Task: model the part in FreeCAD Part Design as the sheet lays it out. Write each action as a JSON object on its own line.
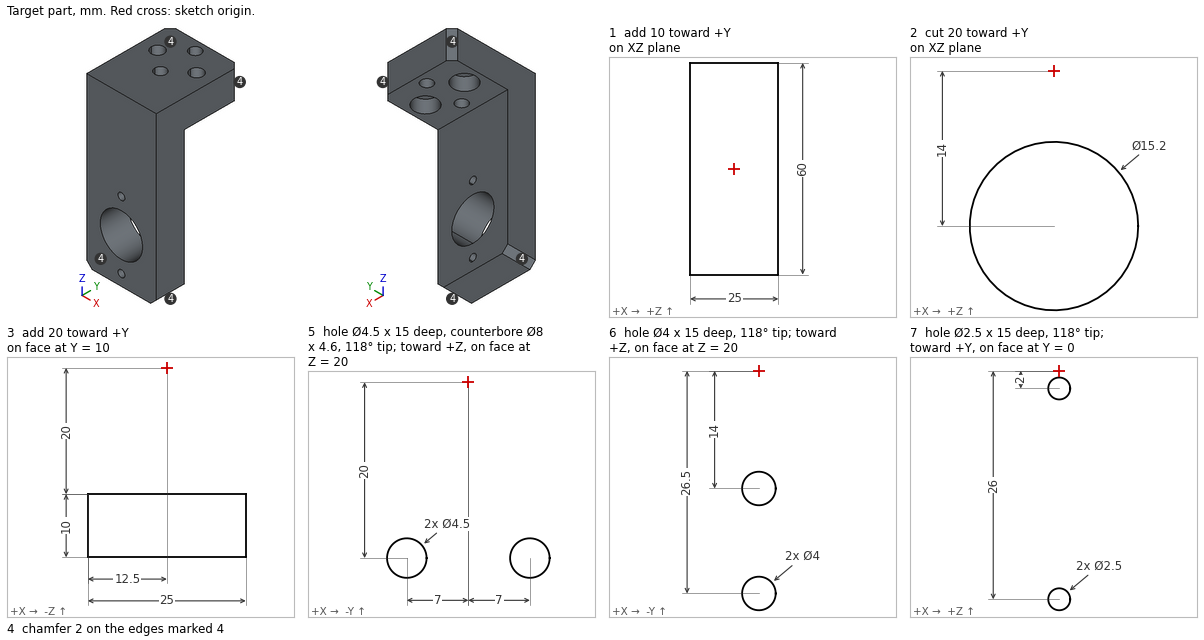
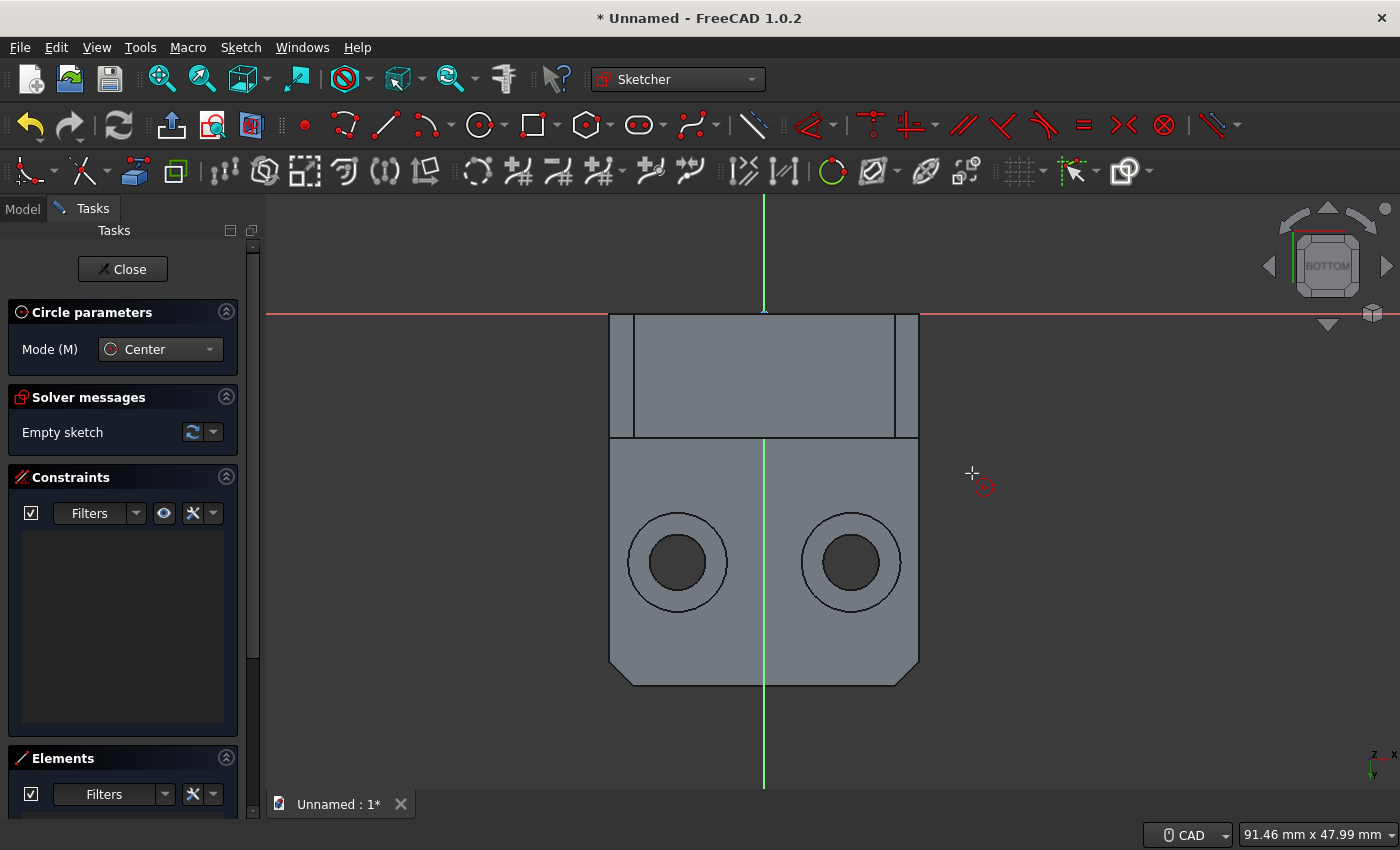
{"action": "left_click", "coordinate": [764, 643]}
{"action": "left_click", "coordinate": [782, 625]}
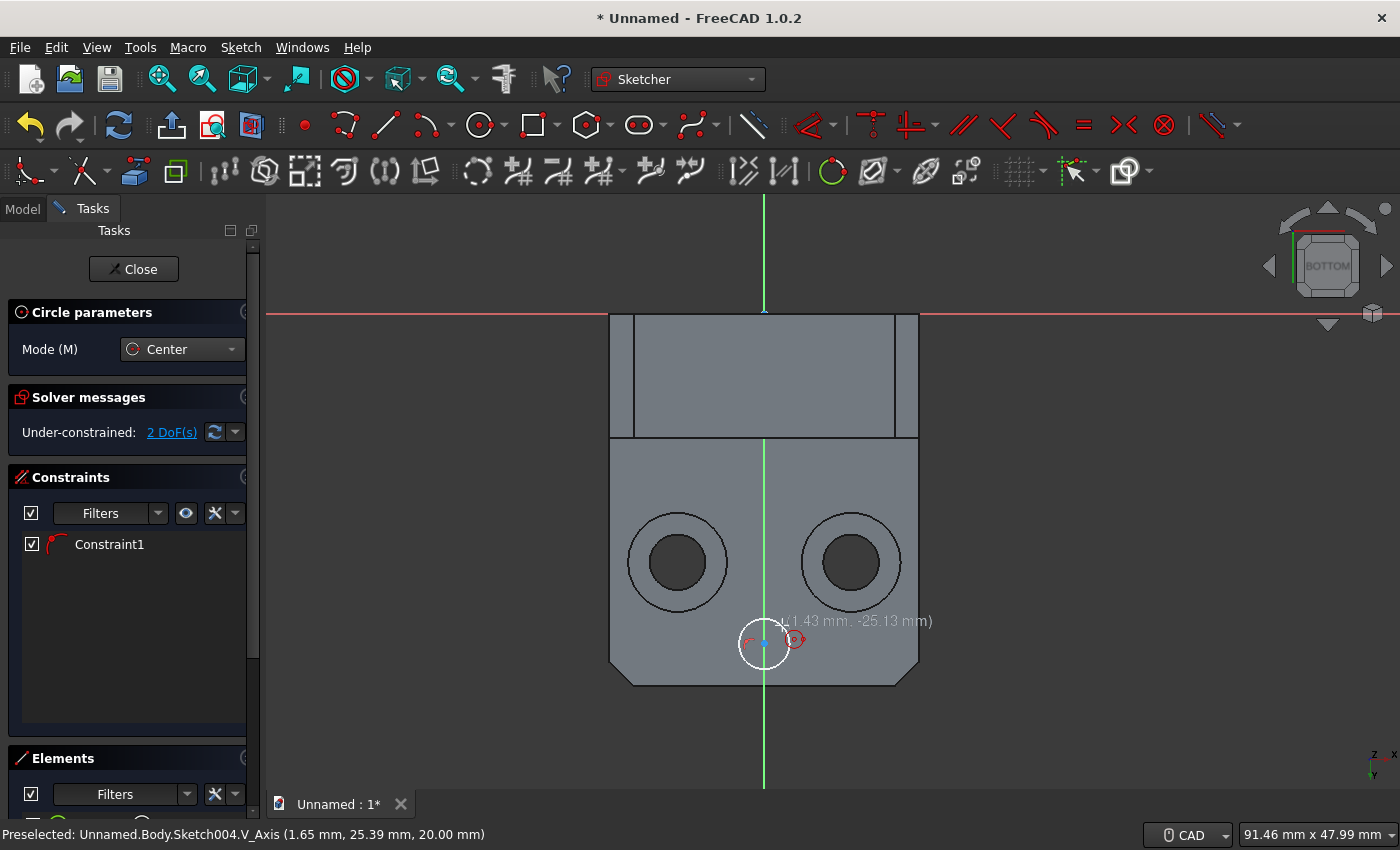
{"action": "left_click", "coordinate": [764, 488]}
{"action": "left_click", "coordinate": [782, 470]}
{"action": "key", "text": "Escape"}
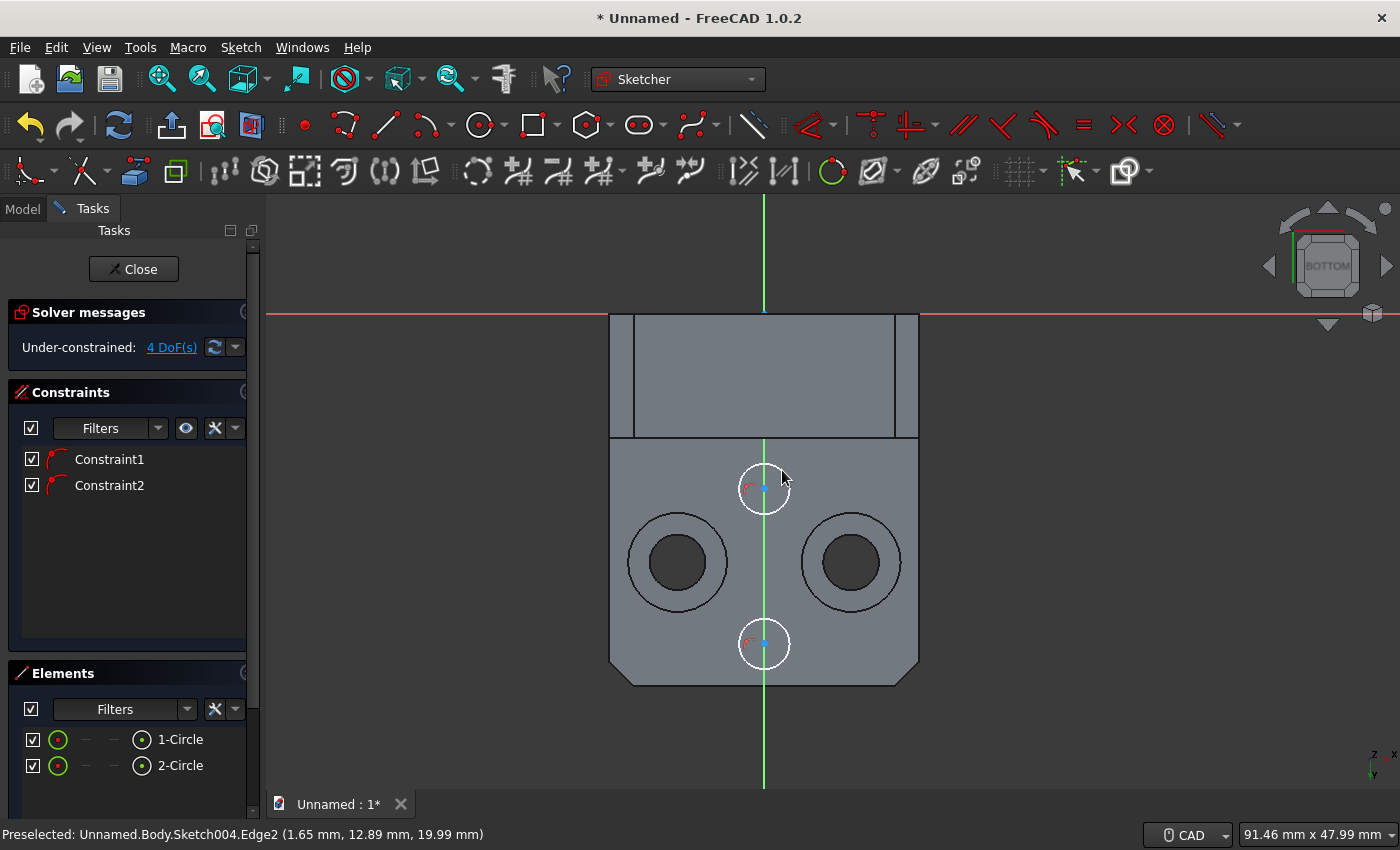
{"action": "left_click", "coordinate": [782, 626]}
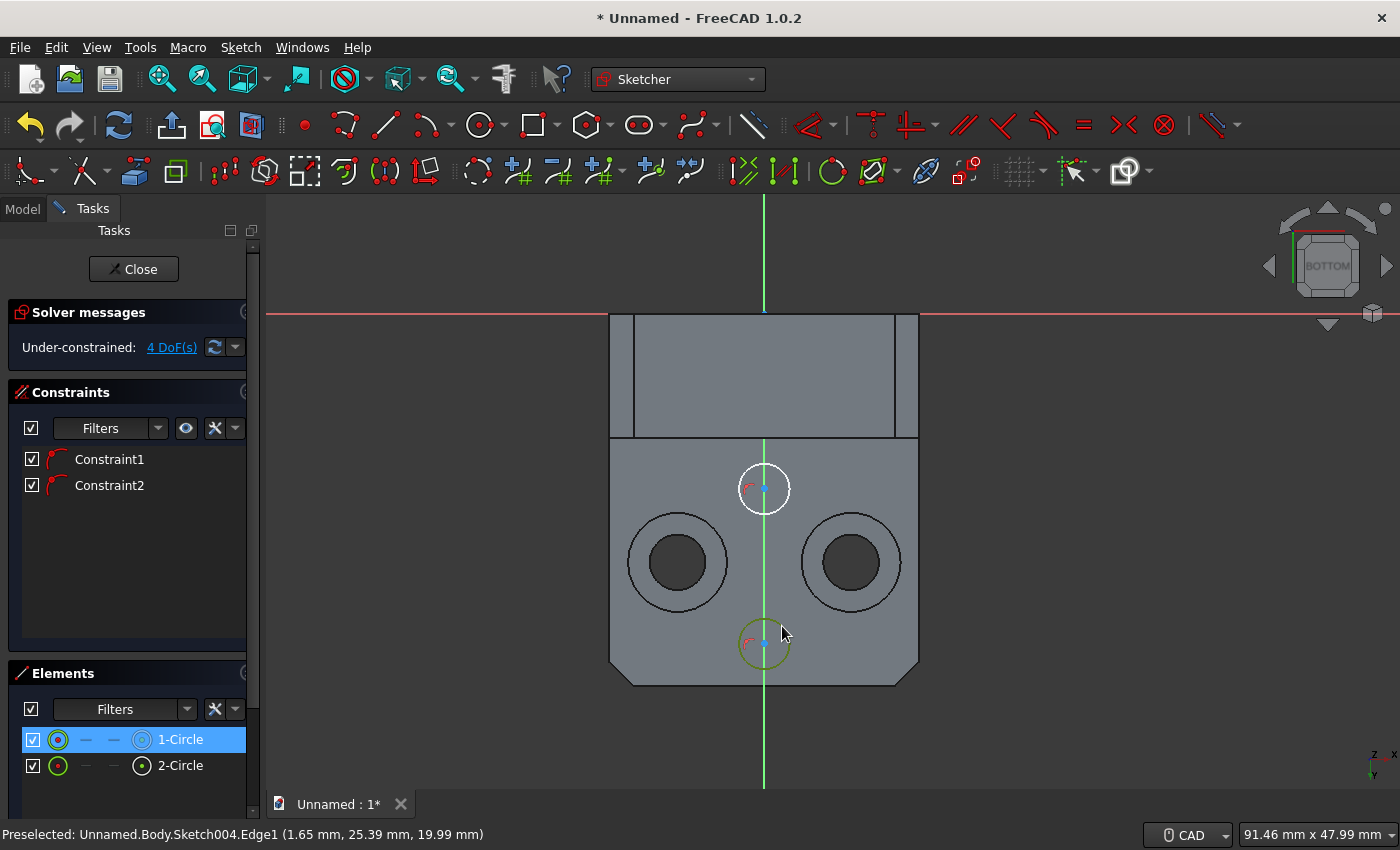
{"action": "left_click", "coordinate": [782, 471]}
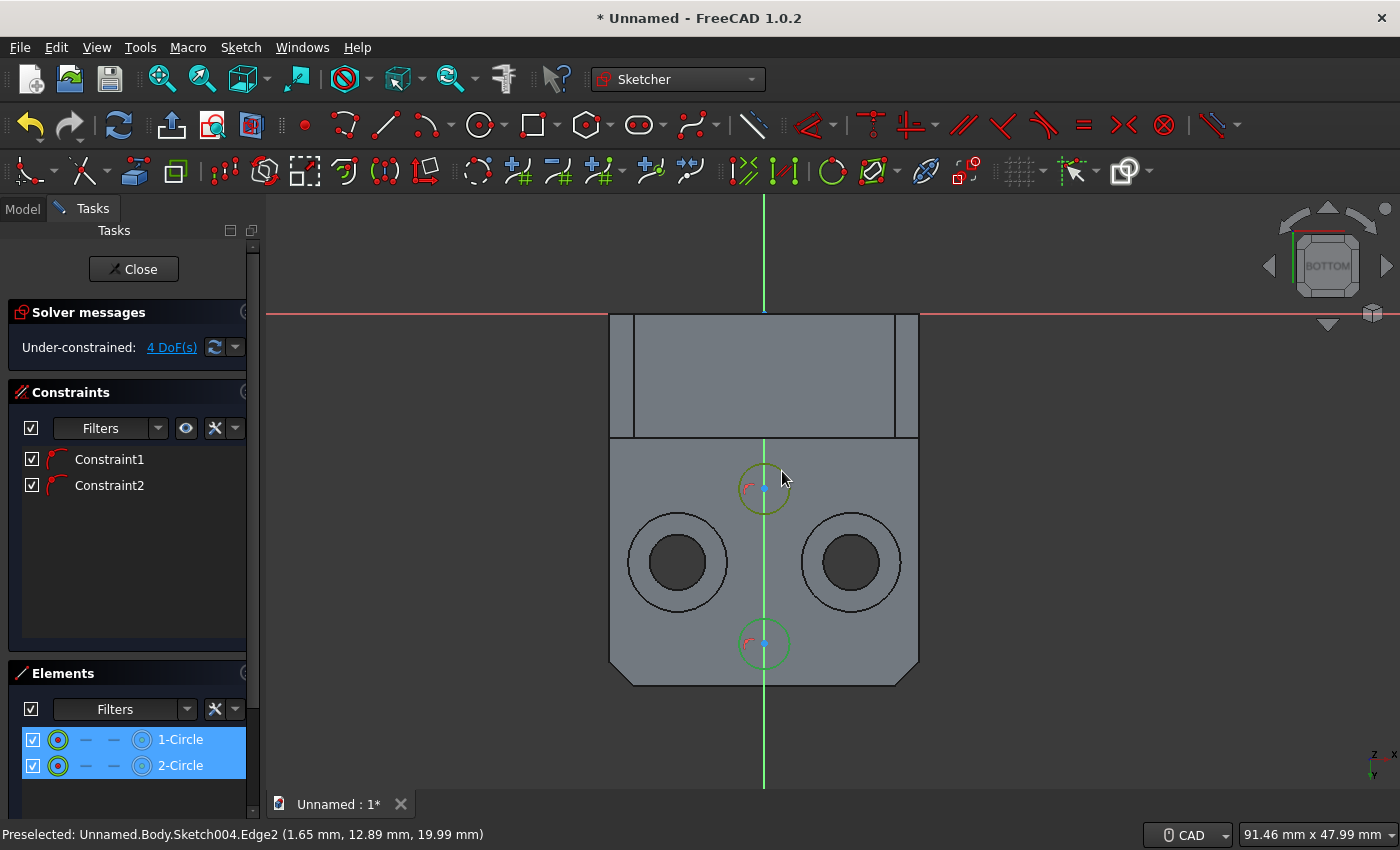
{"action": "key", "text": "e"}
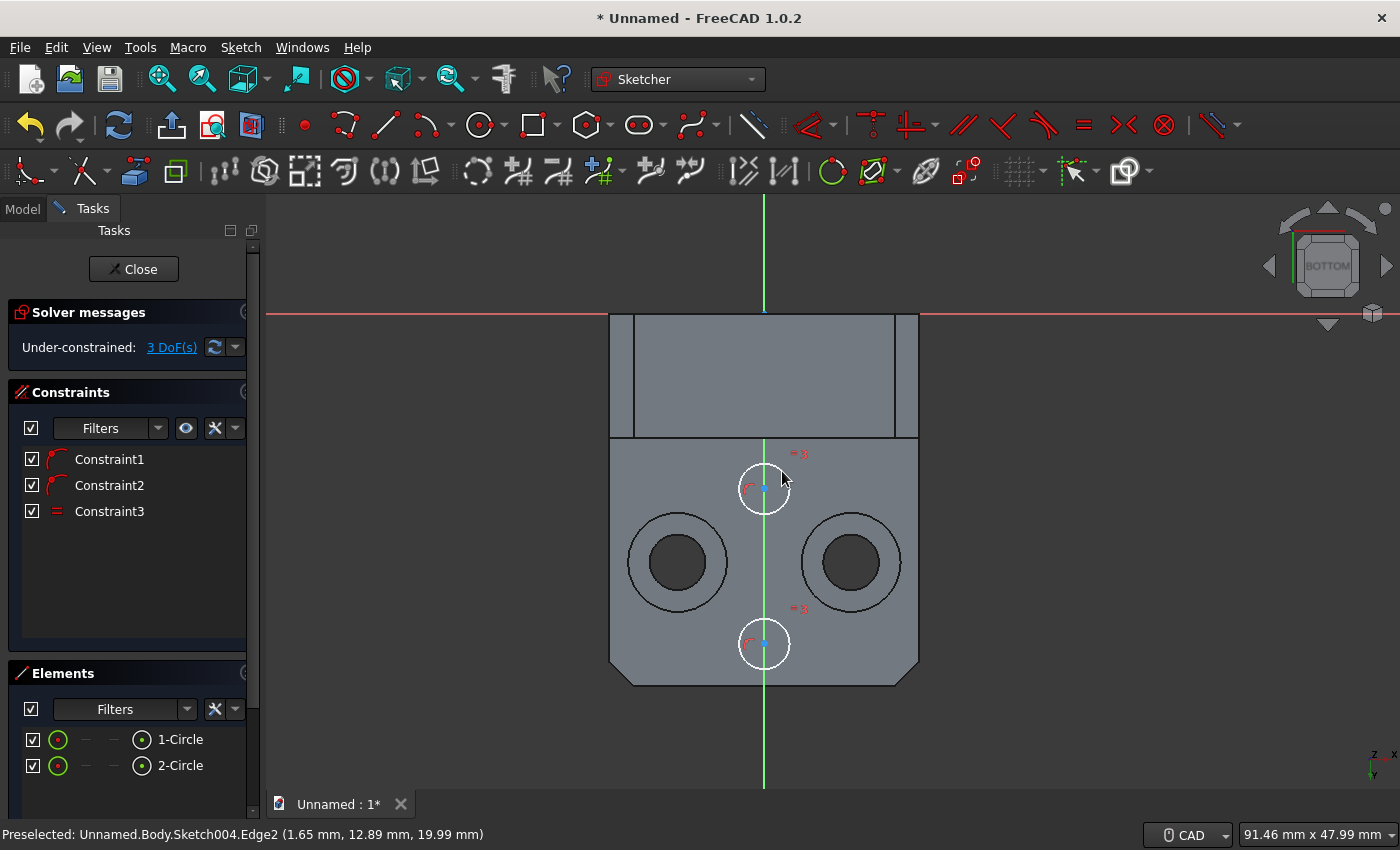
{"action": "key", "text": "d"}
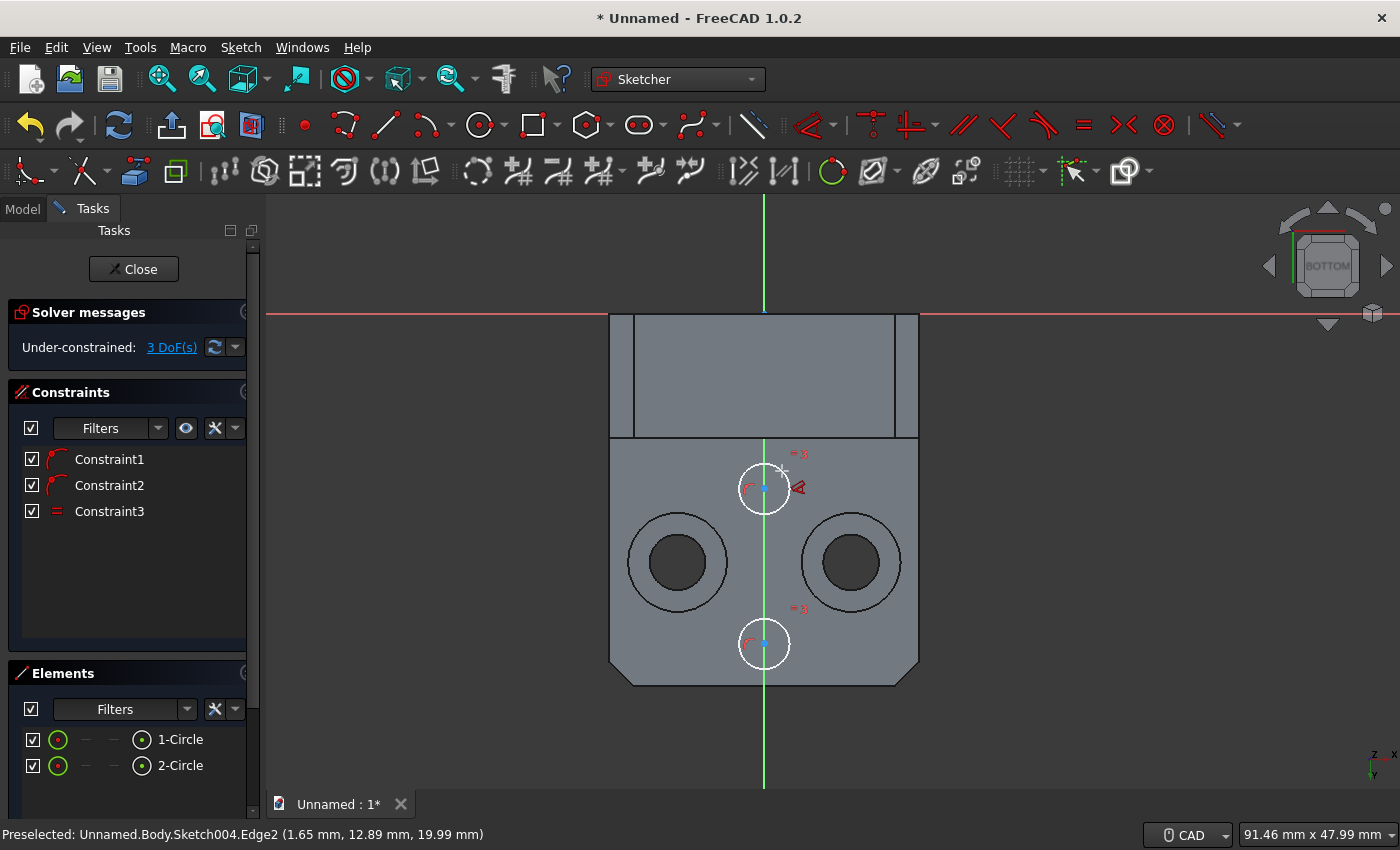
{"action": "left_click", "coordinate": [782, 626]}
{"action": "left_click", "coordinate": [804, 603]}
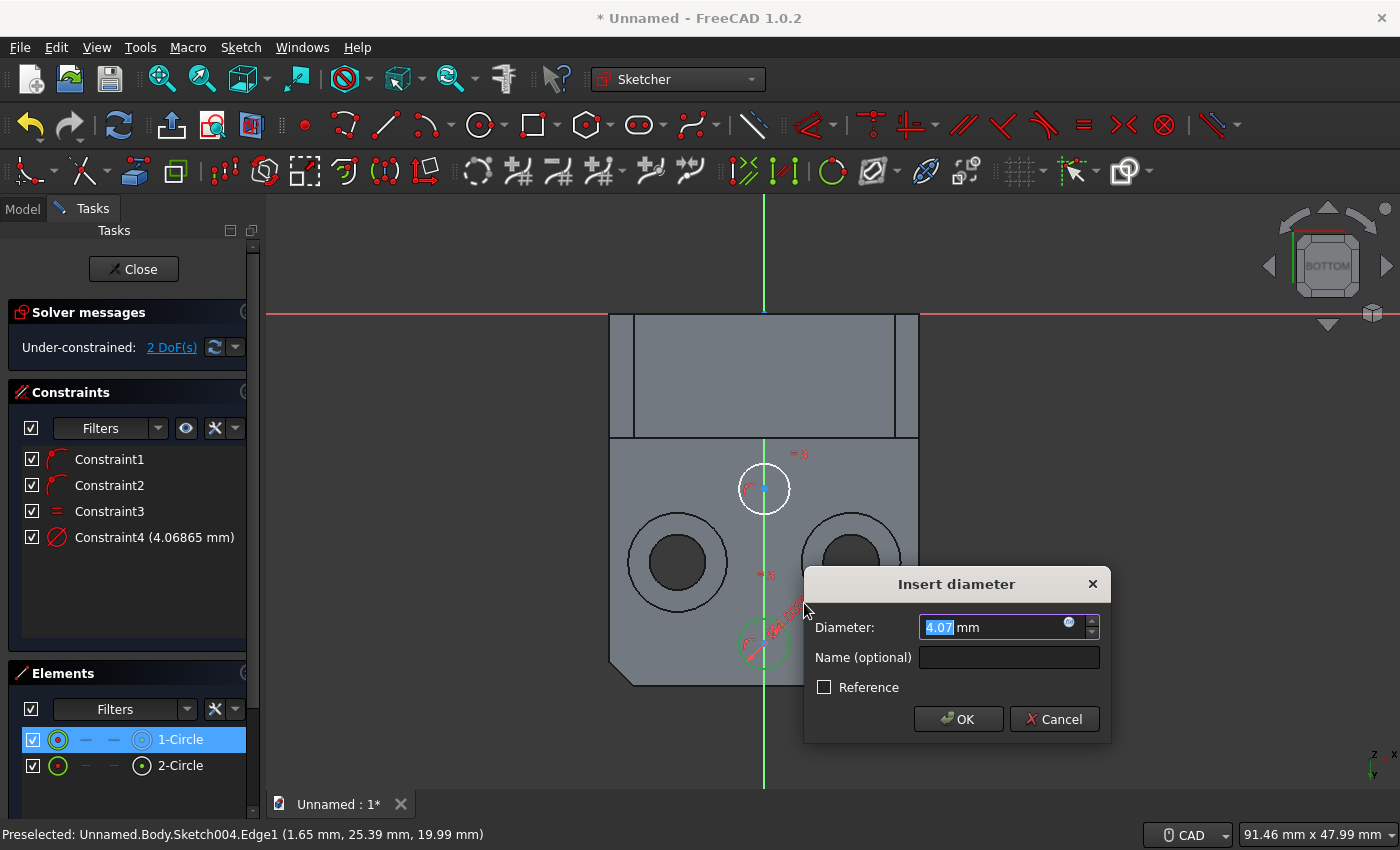
{"action": "type", "text": "4"}
{"action": "key", "text": "Return"}